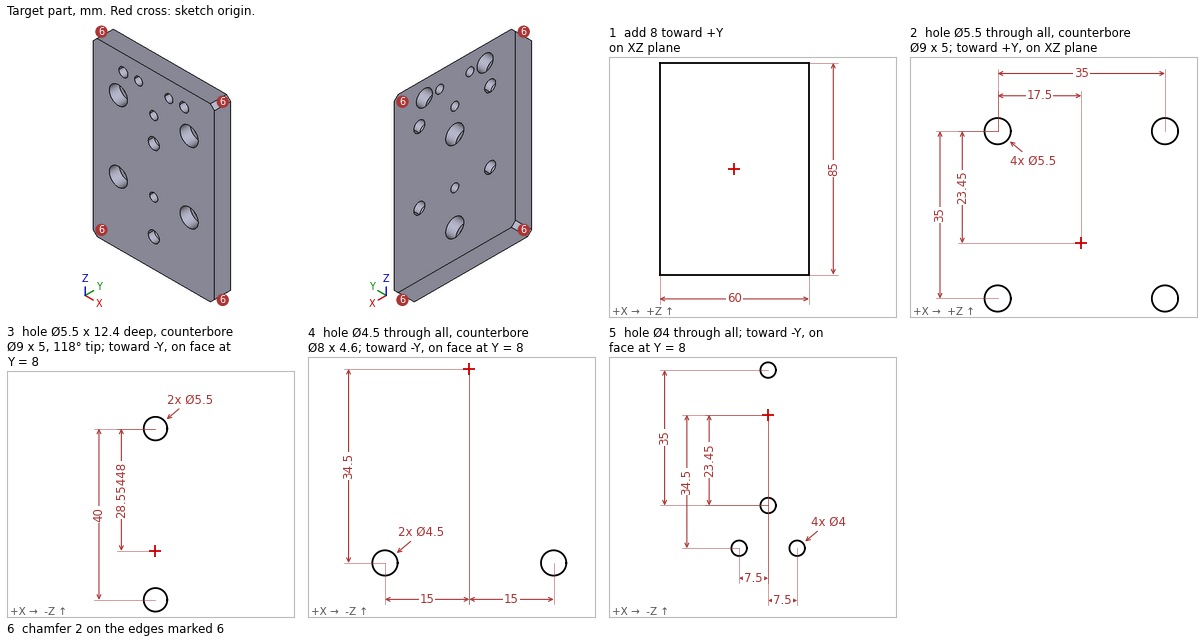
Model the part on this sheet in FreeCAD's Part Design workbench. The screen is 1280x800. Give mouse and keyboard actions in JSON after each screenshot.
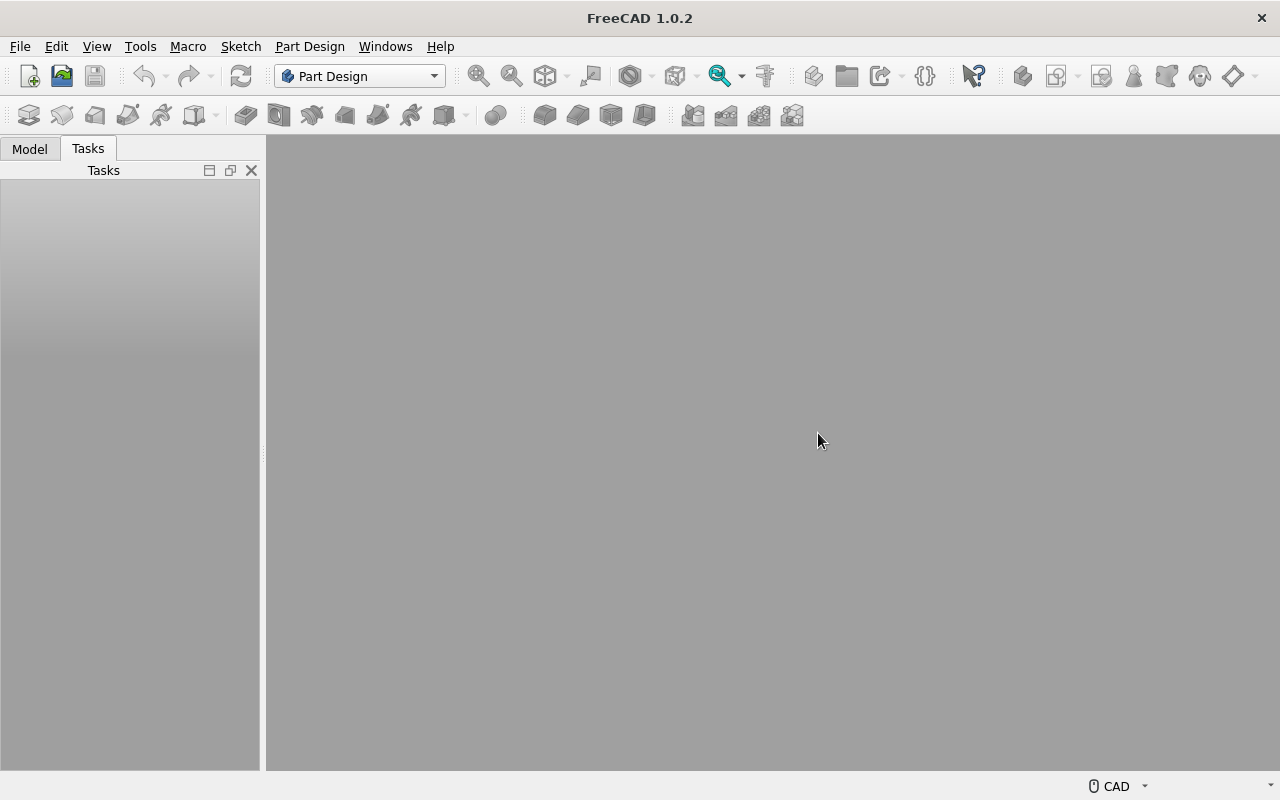
{"action": "key", "text": "ctrl+n"}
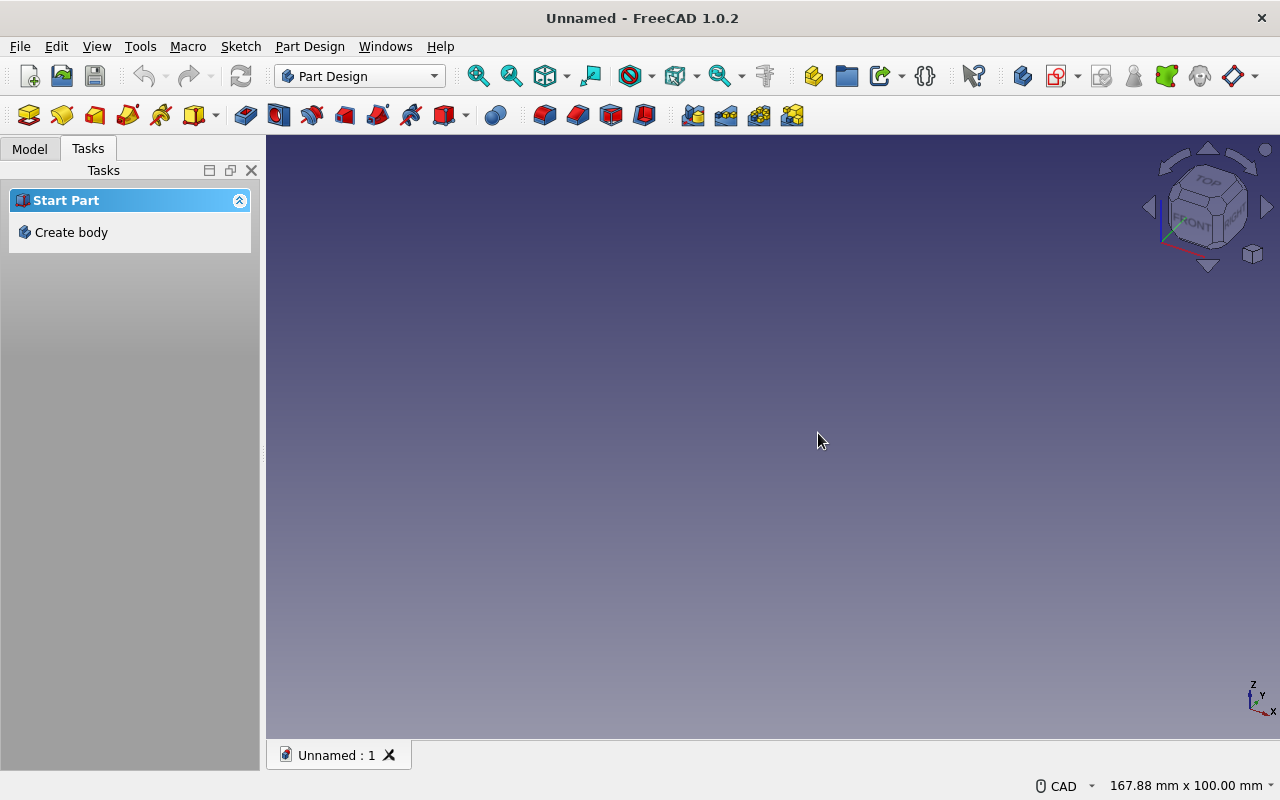
{"action": "left_click", "coordinate": [1056, 76]}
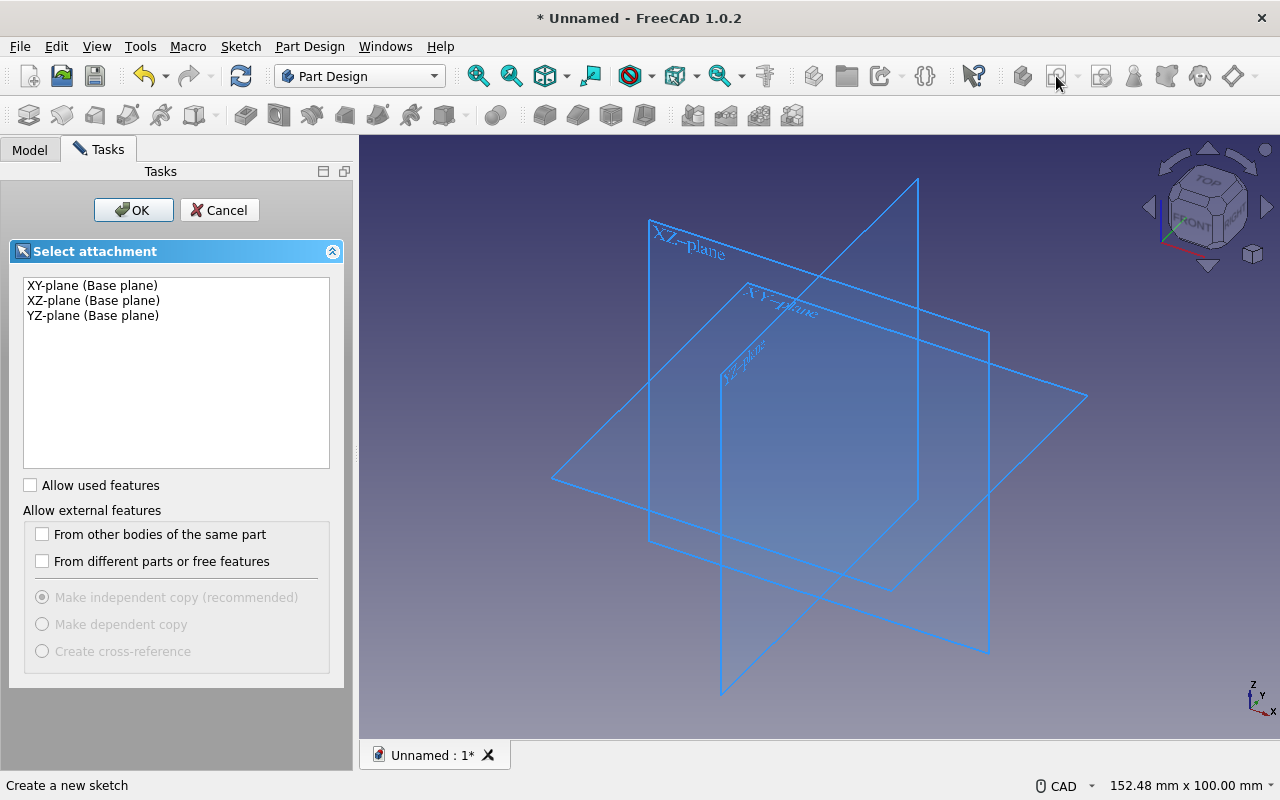
{"action": "left_click", "coordinate": [84, 300]}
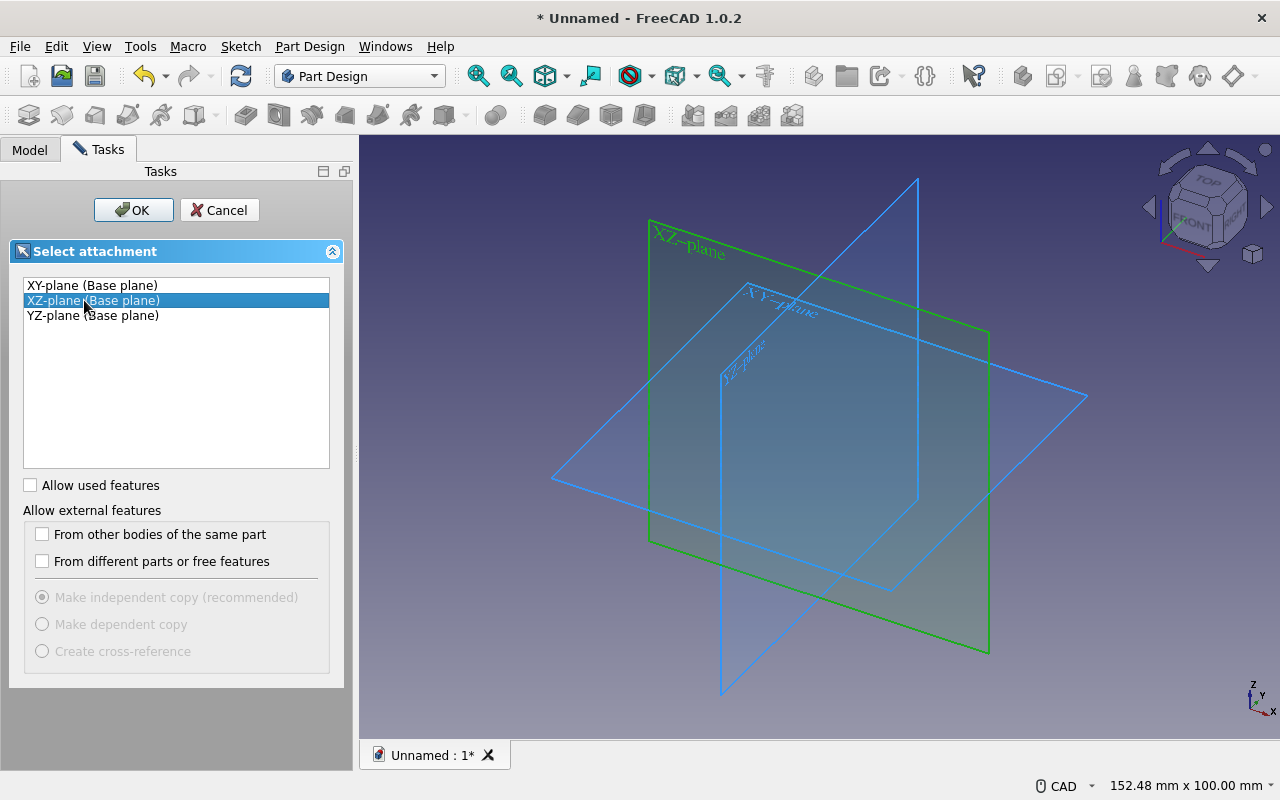
{"action": "left_click", "coordinate": [134, 210]}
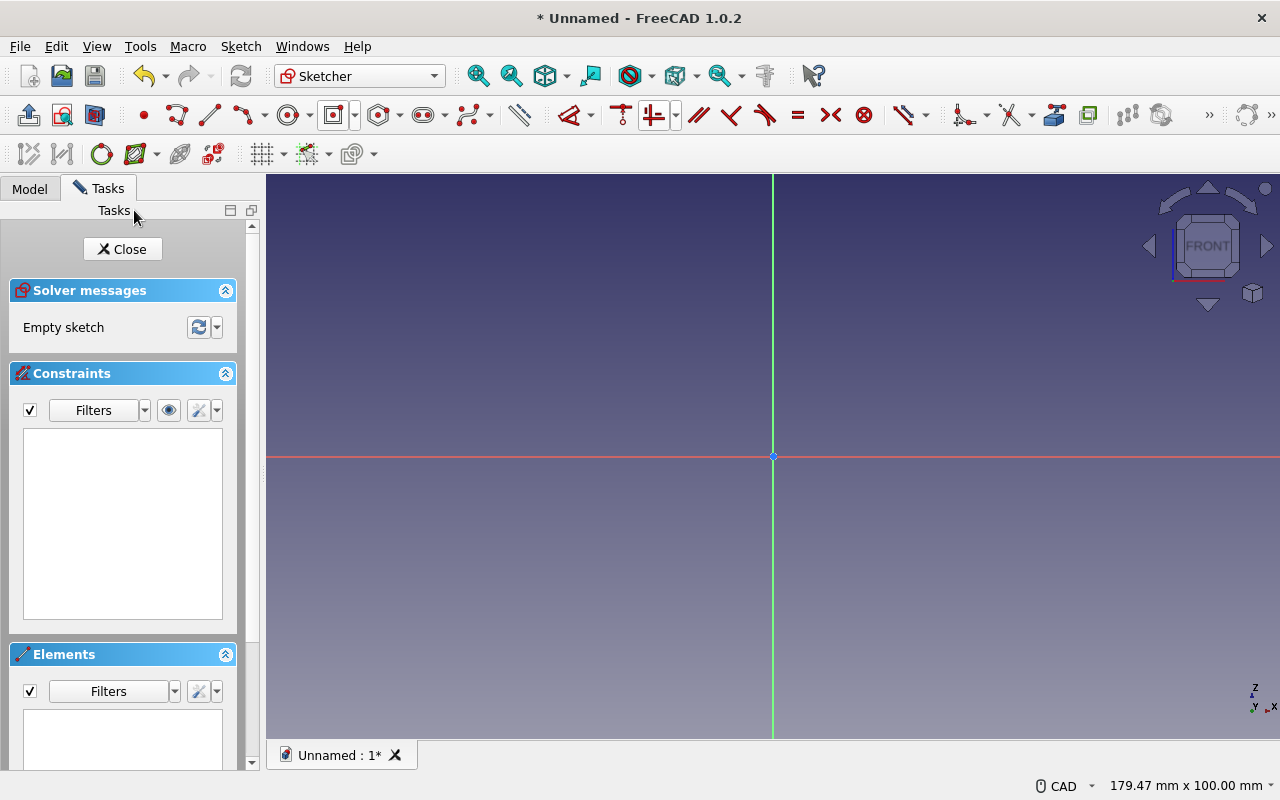
{"action": "scroll", "coordinate": [395, 456], "scroll_direction": "down", "scroll_amount": 1}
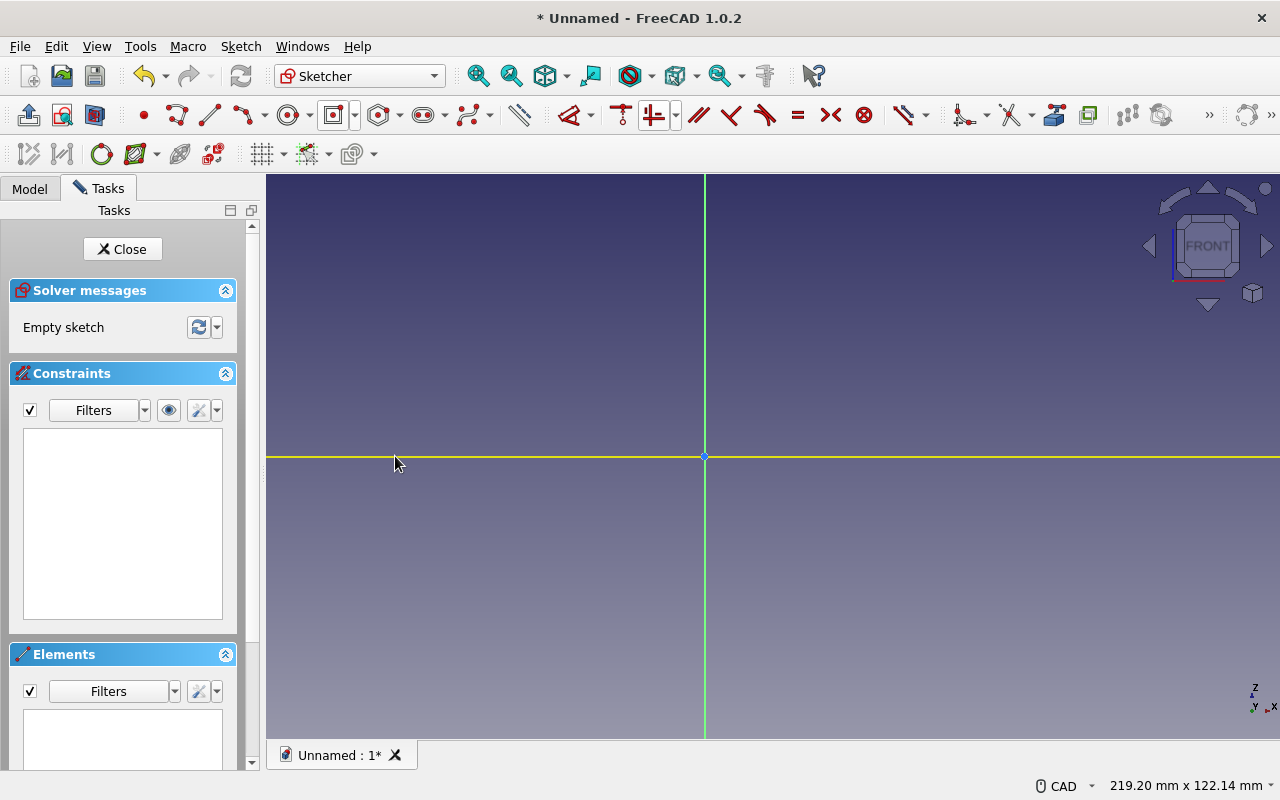
{"action": "left_click", "coordinate": [332, 116]}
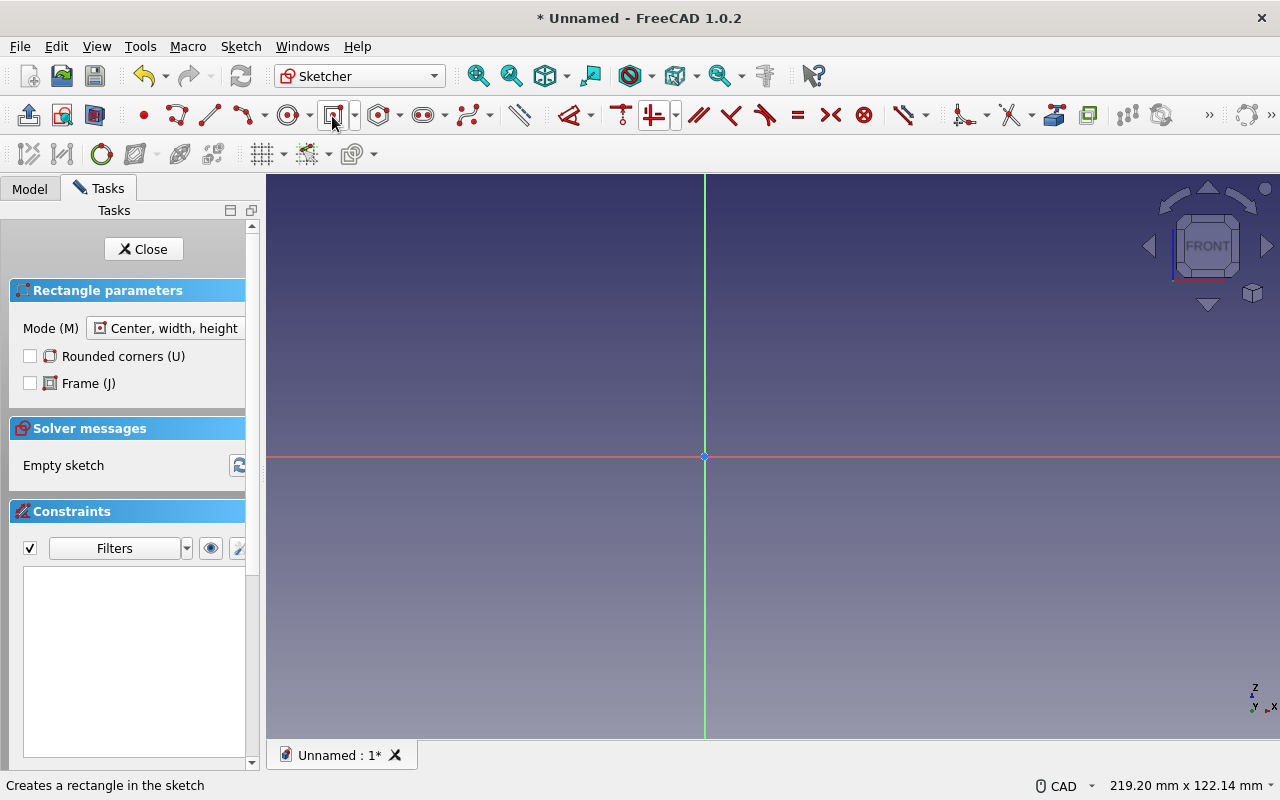
{"action": "left_click", "coordinate": [705, 456]}
{"action": "left_click", "coordinate": [843, 260]}
{"action": "key", "text": "Escape"}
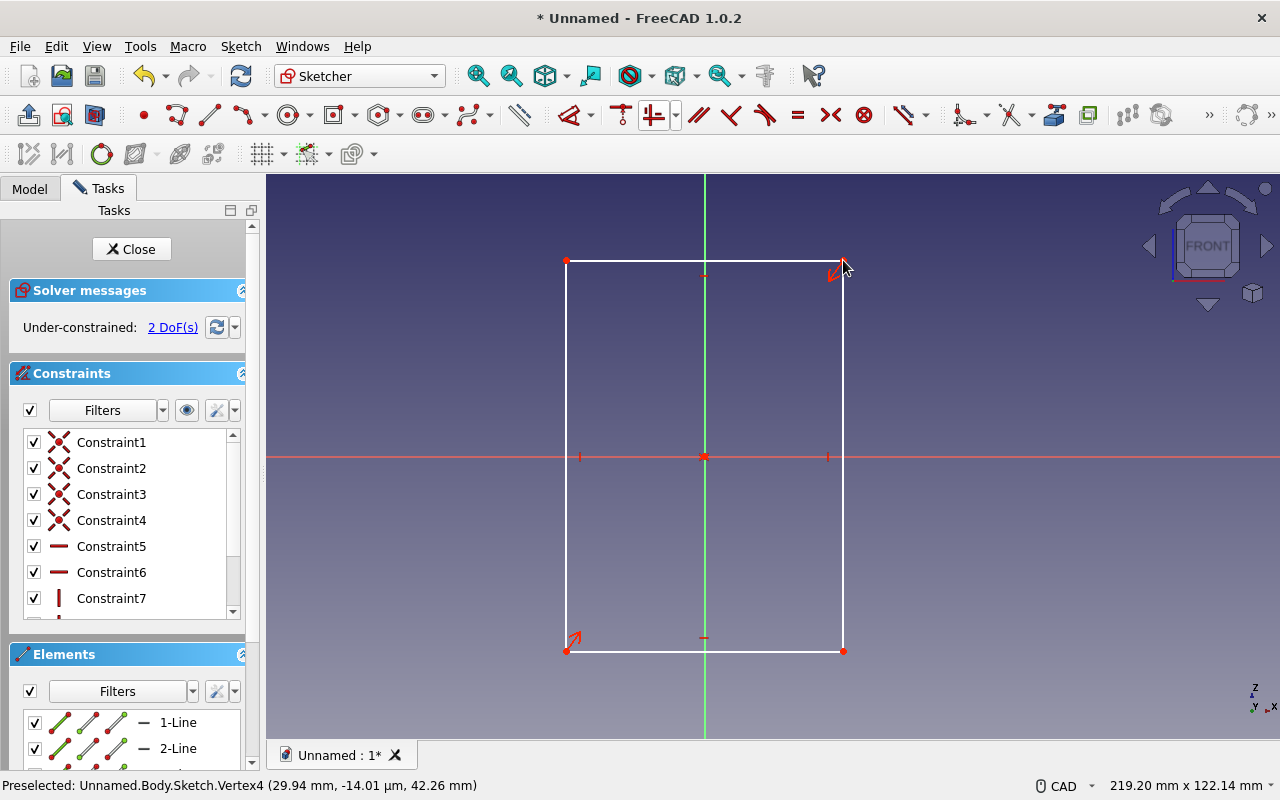
{"action": "left_click", "coordinate": [649, 652]}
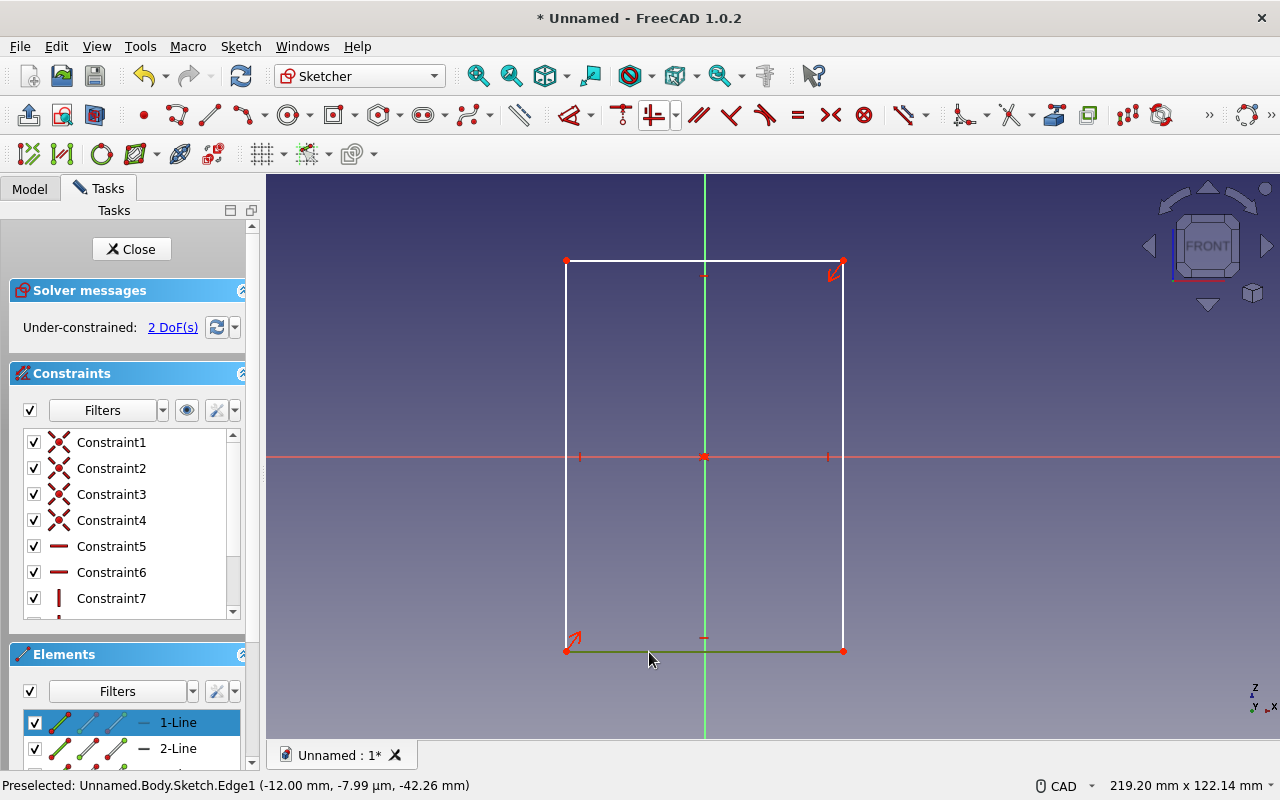
{"action": "left_click", "coordinate": [590, 116]}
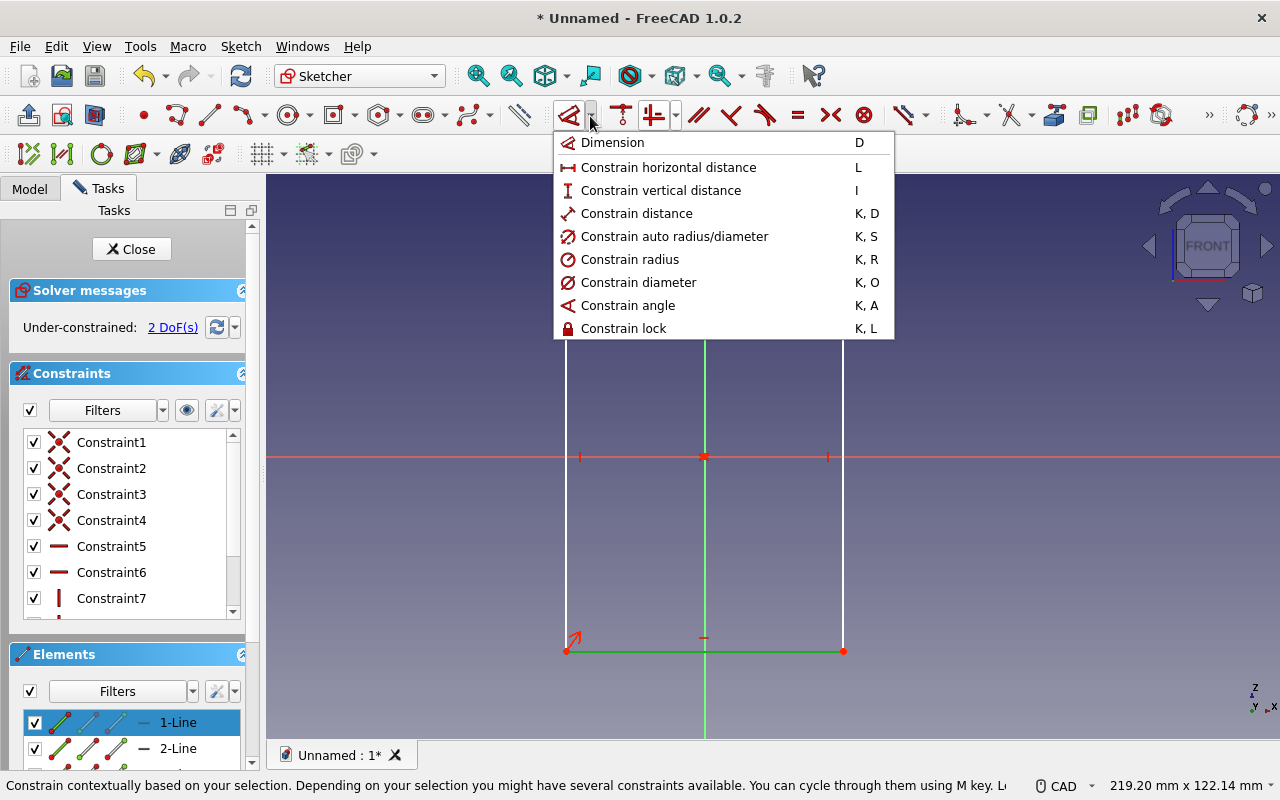
{"action": "left_click", "coordinate": [724, 168]}